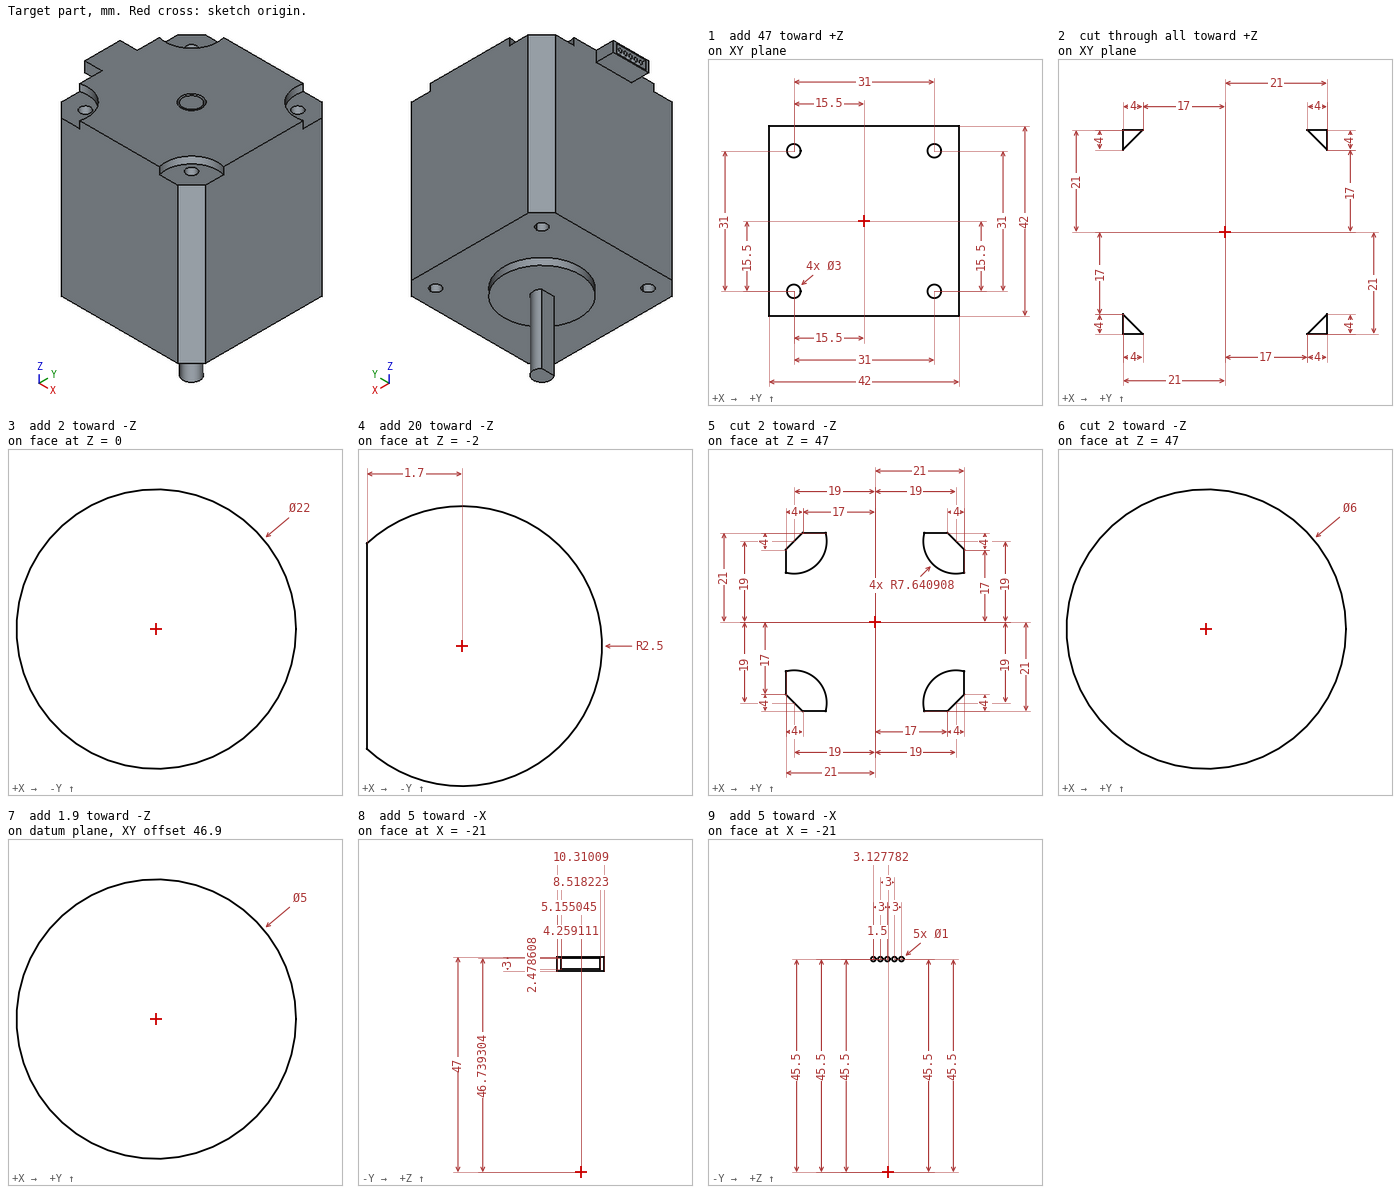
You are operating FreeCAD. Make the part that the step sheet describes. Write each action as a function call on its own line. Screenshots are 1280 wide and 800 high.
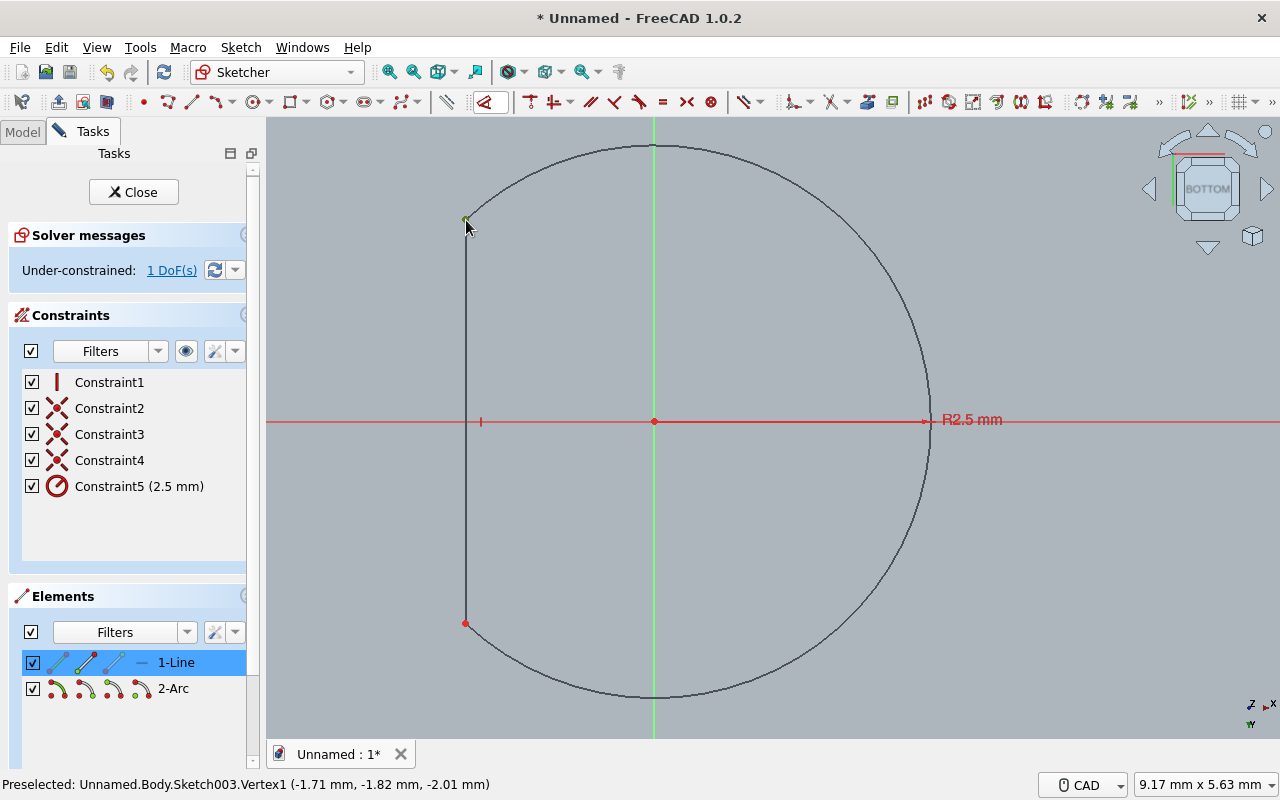
key(l)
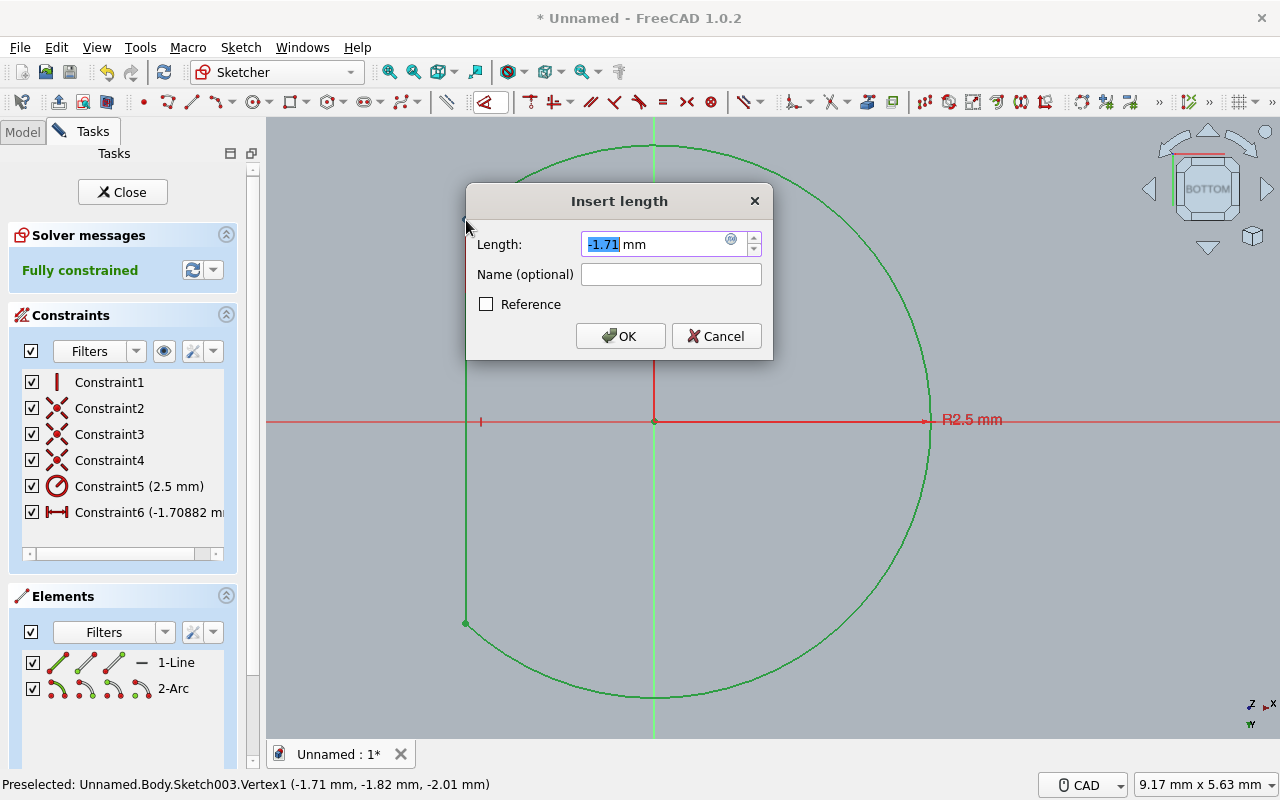
text(-1.7)
key(Return)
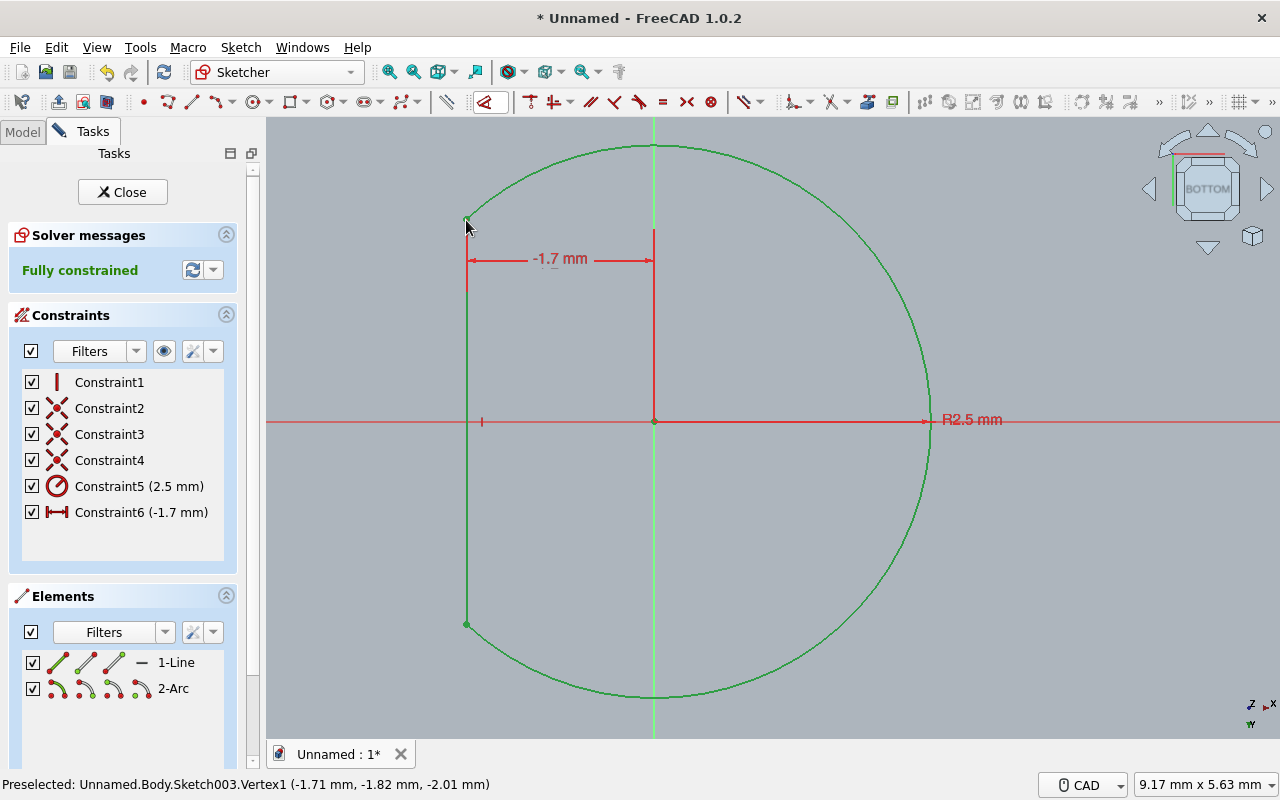
click(123, 192)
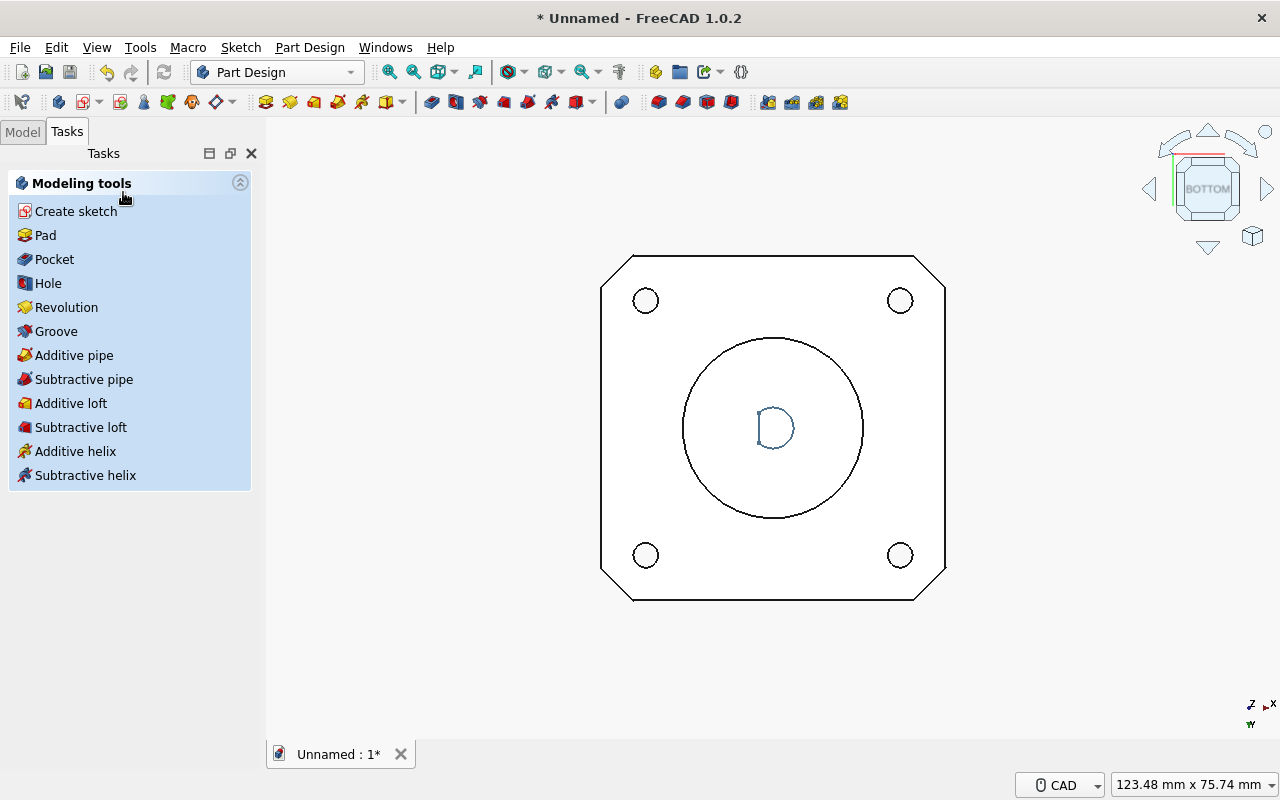
click(266, 102)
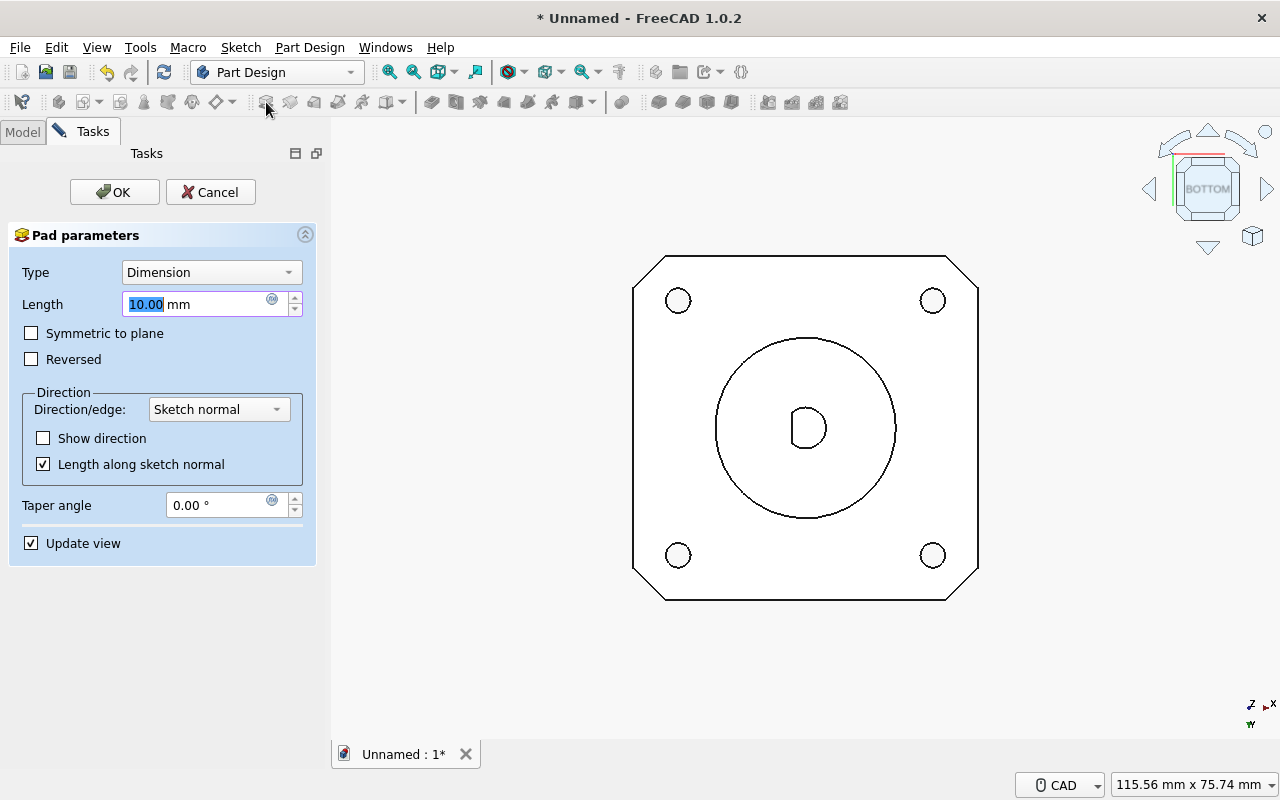
text(20)
key(Tab)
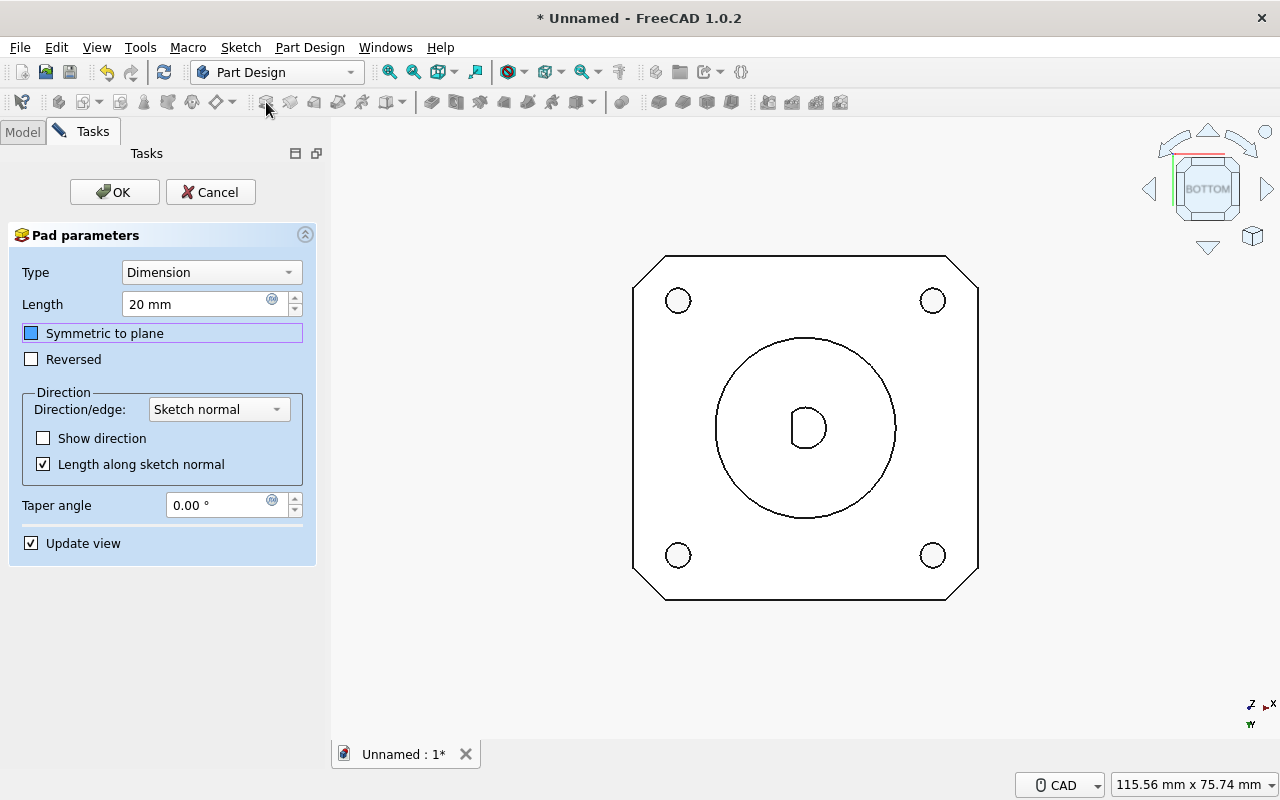
click(115, 192)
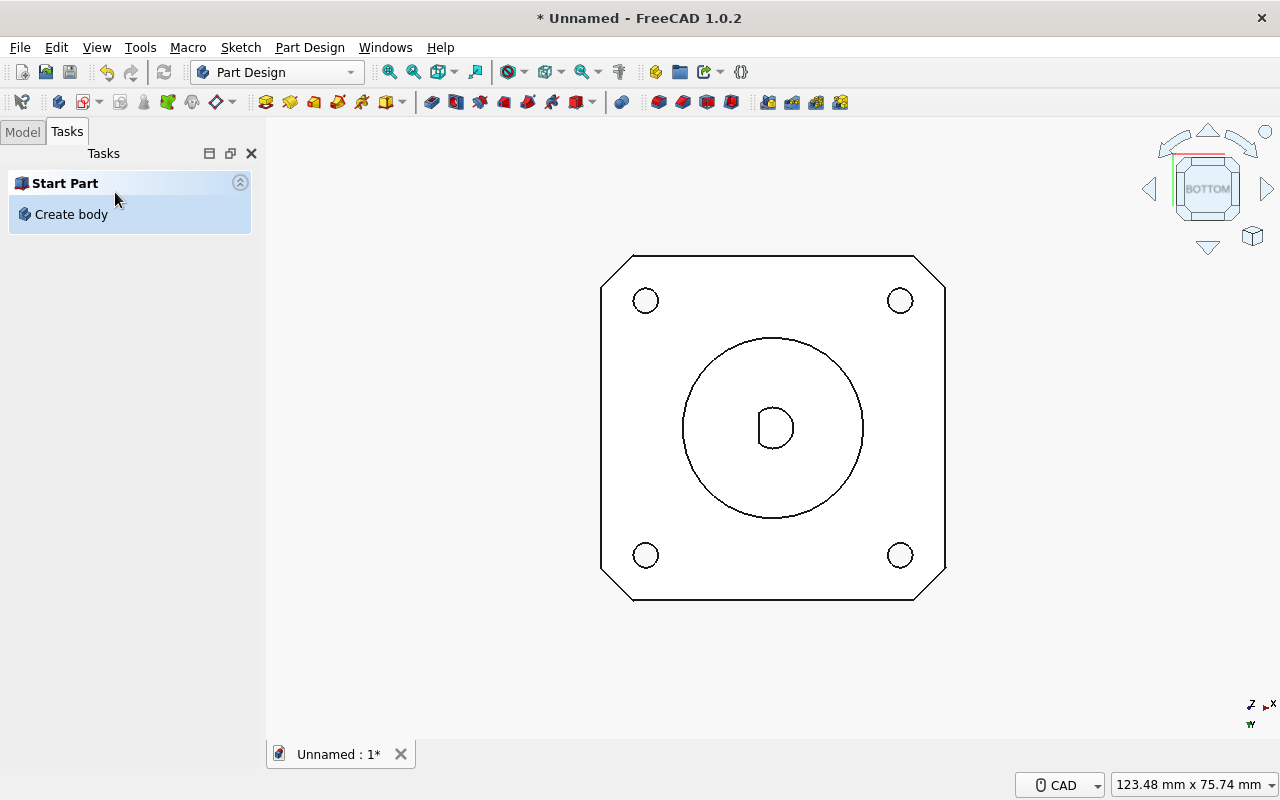
key(0)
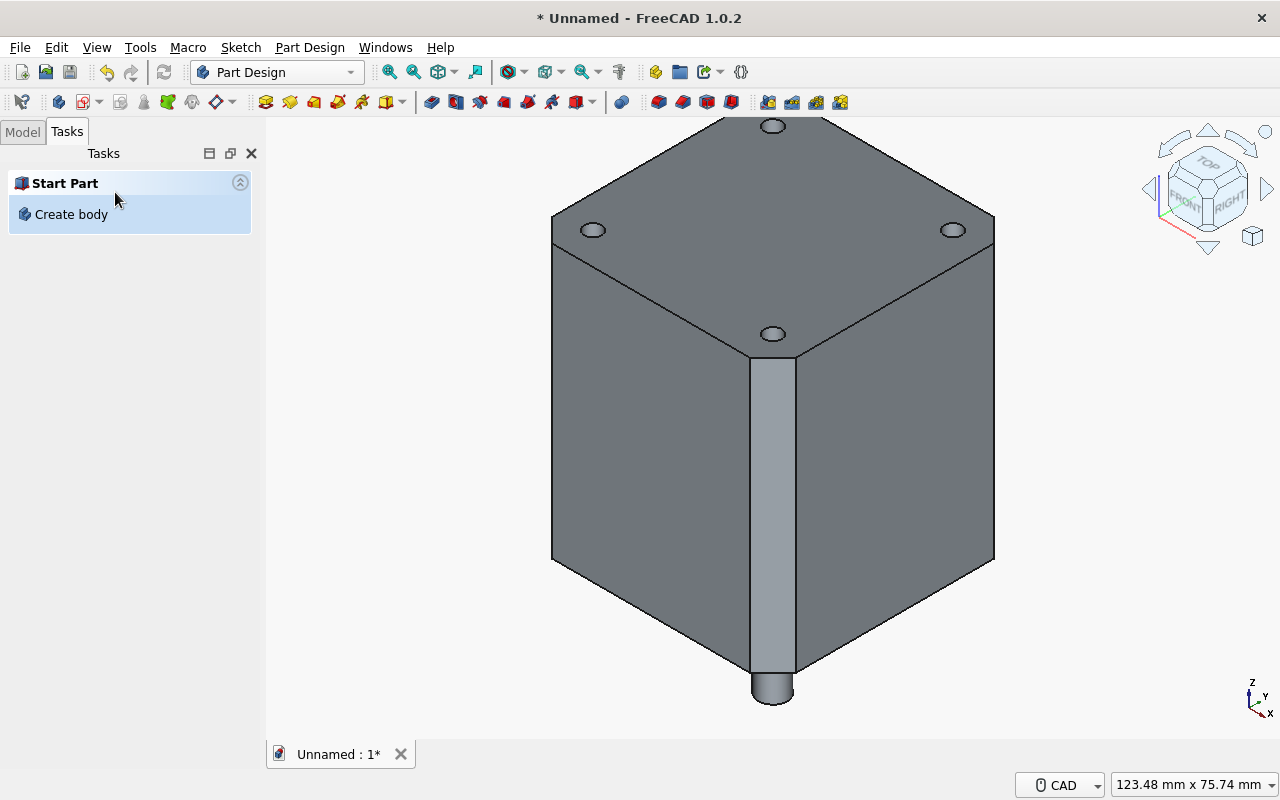
click(390, 72)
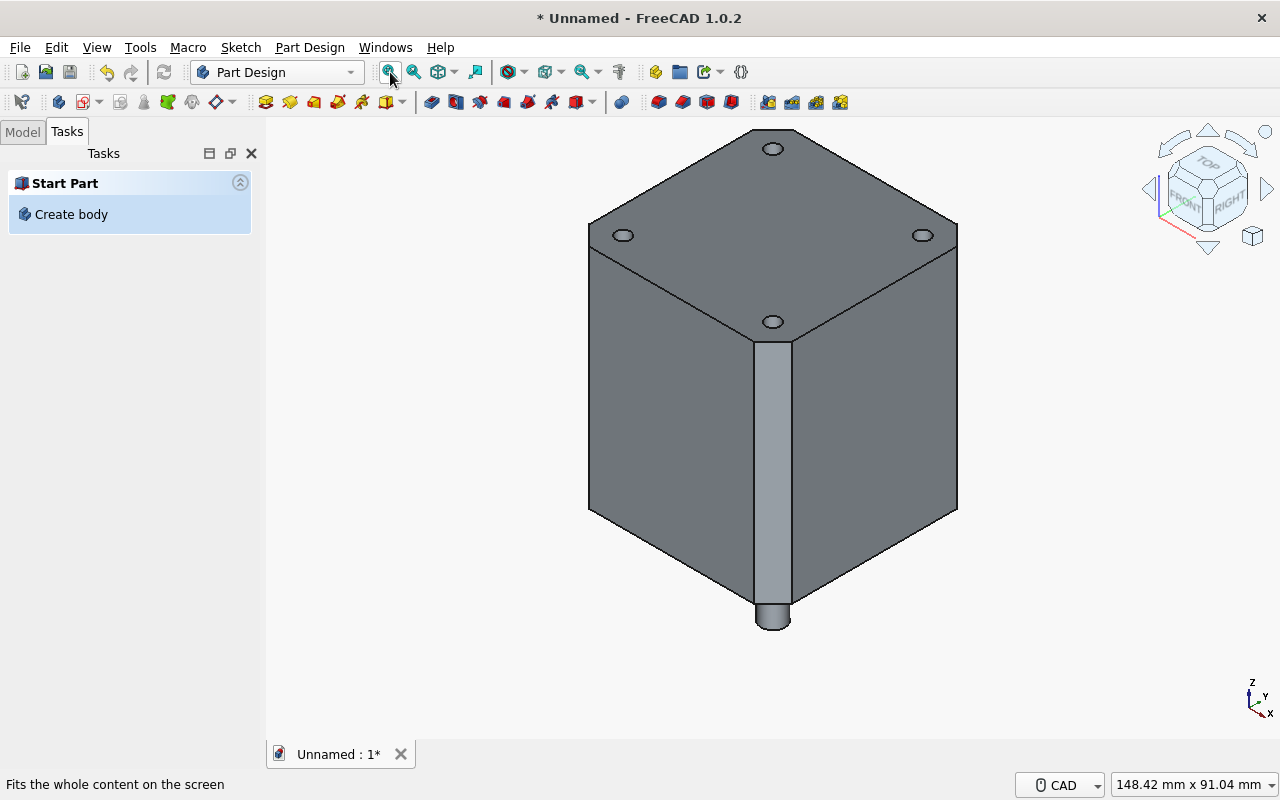
click(773, 235)